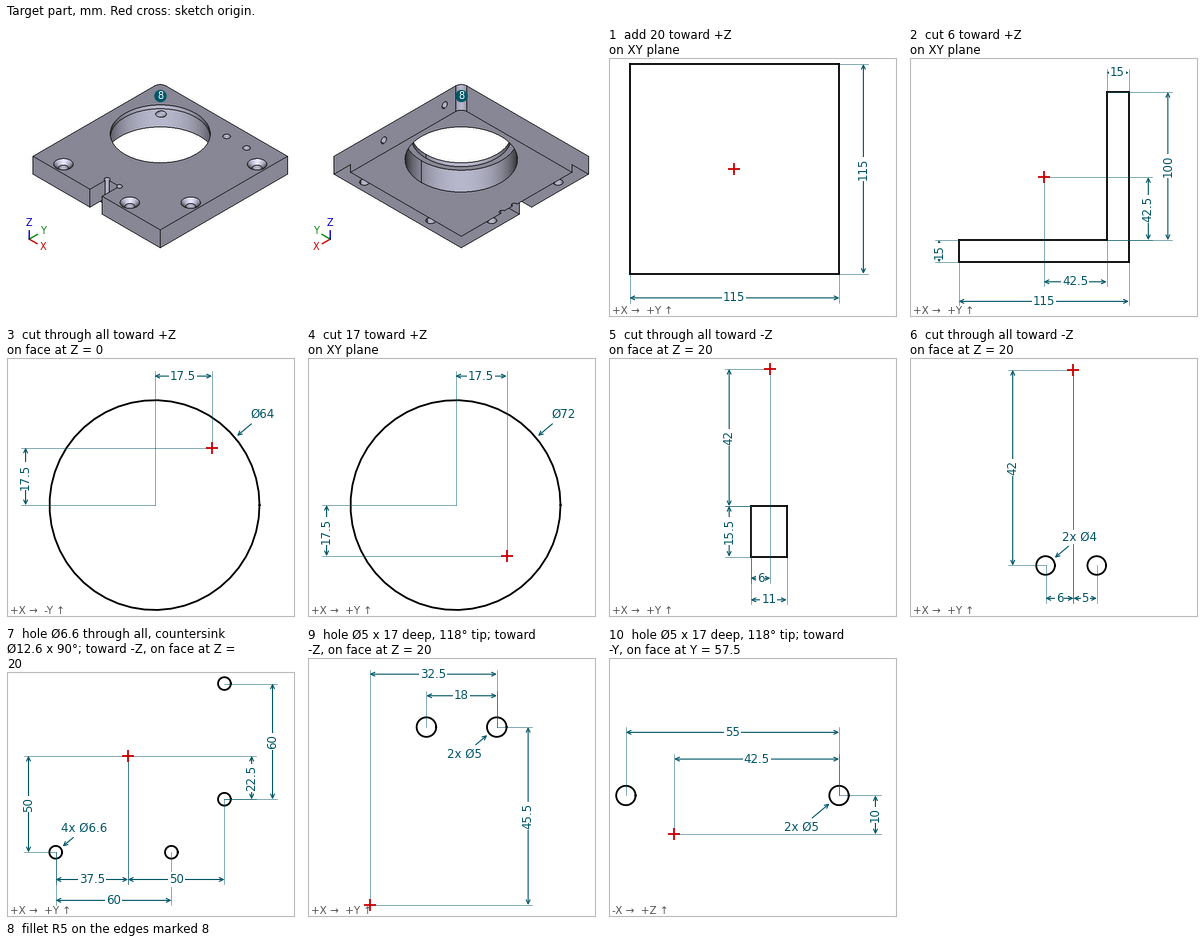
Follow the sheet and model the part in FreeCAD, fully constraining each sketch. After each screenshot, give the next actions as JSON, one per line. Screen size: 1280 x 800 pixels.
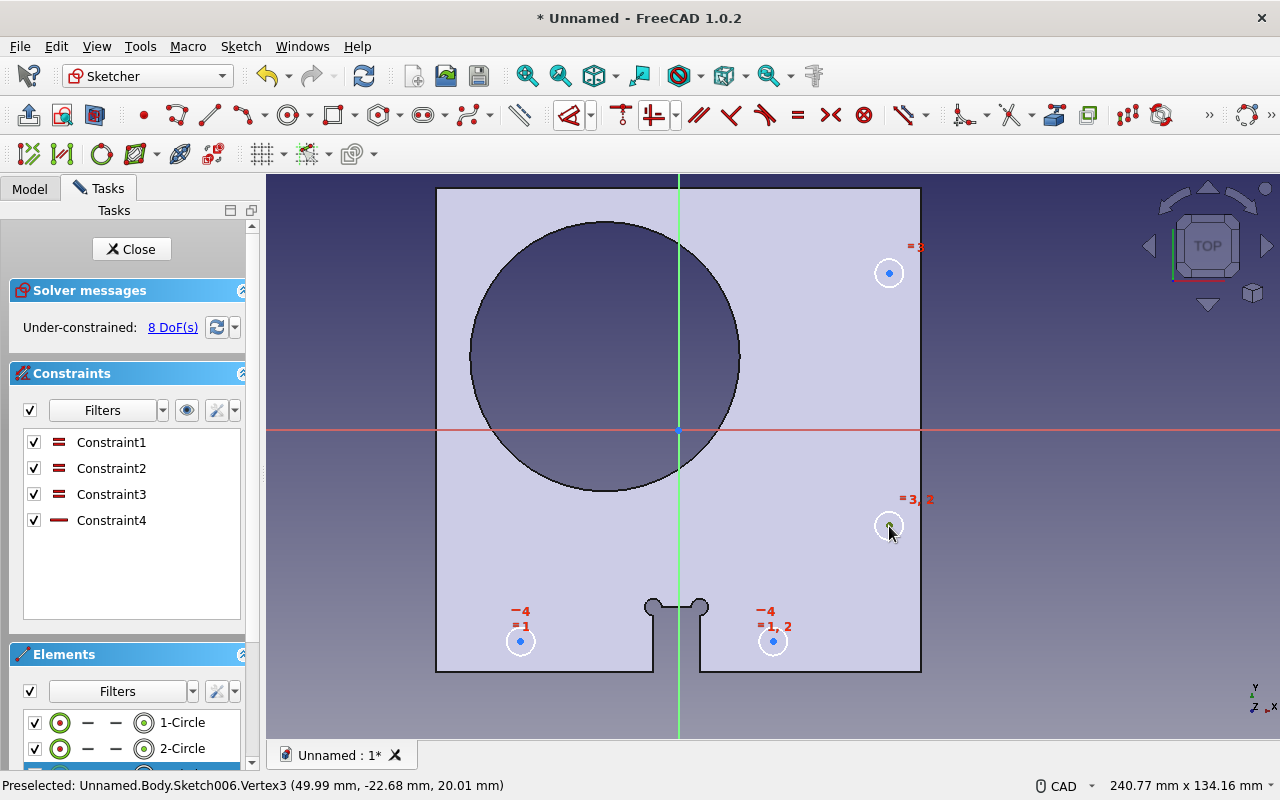
{"action": "left_click", "coordinate": [889, 273]}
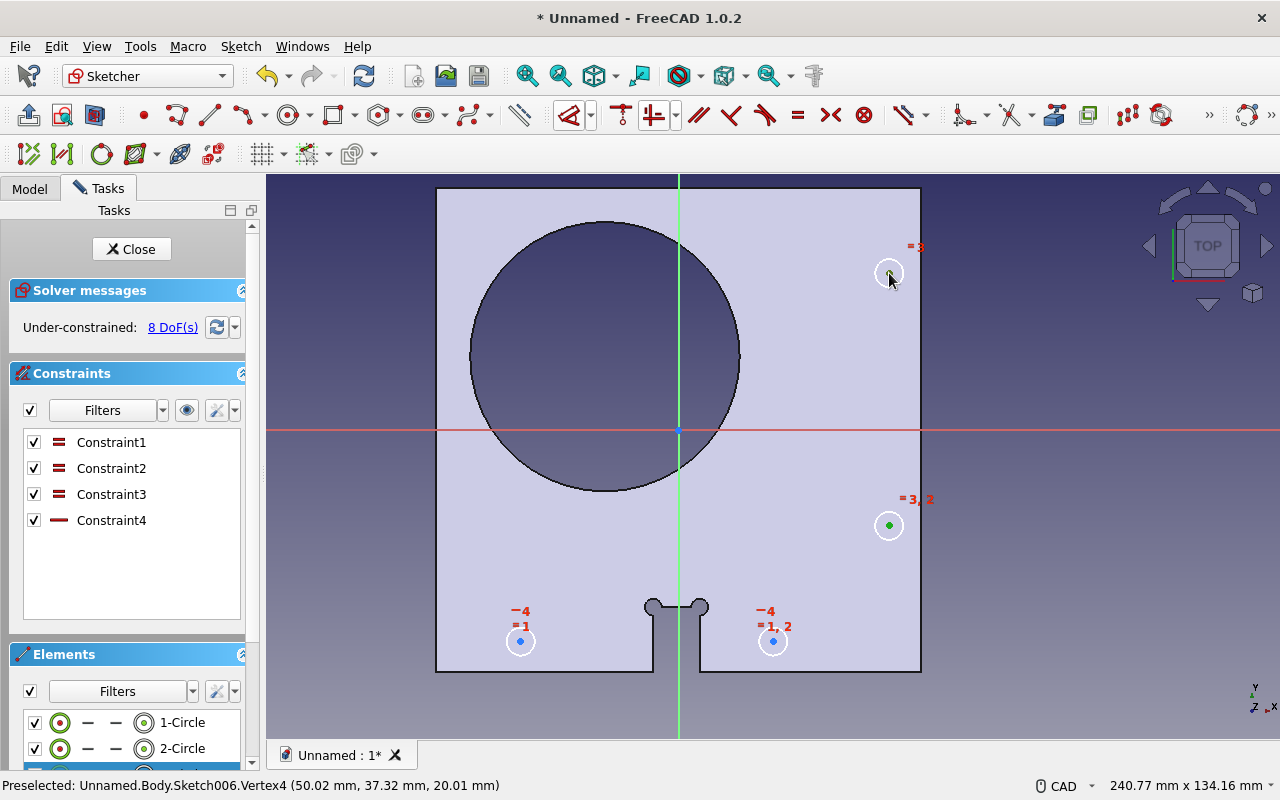
{"action": "key", "text": "v"}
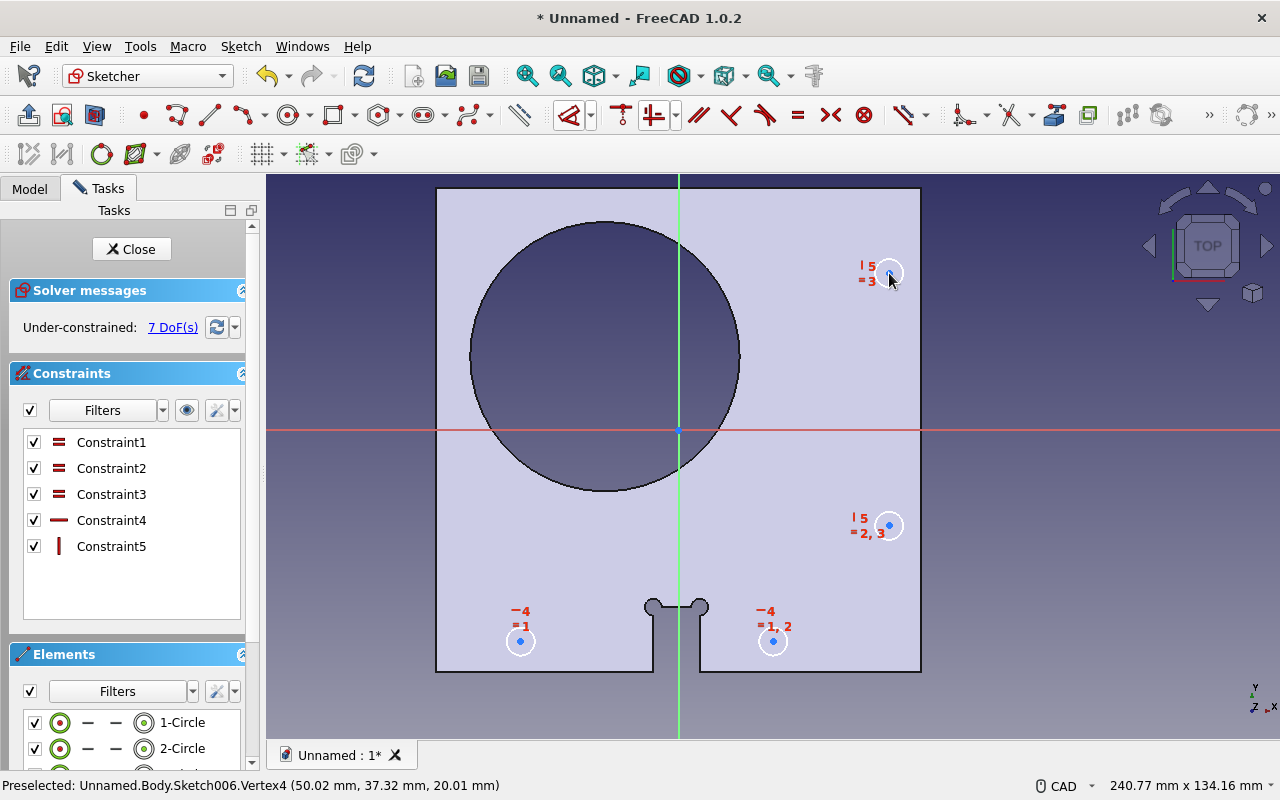
{"action": "scroll", "coordinate": [531, 632], "scroll_direction": "up", "scroll_amount": 2}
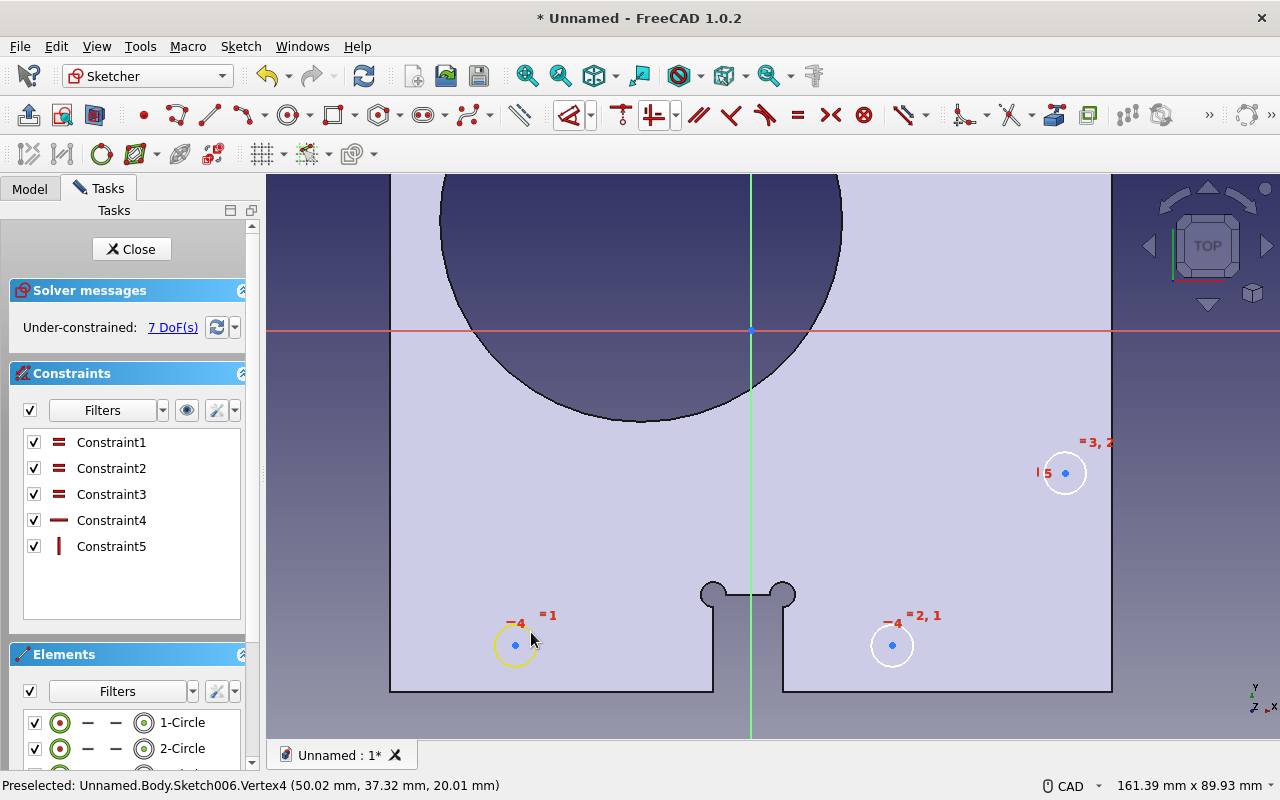
{"action": "left_click", "coordinate": [530, 631]}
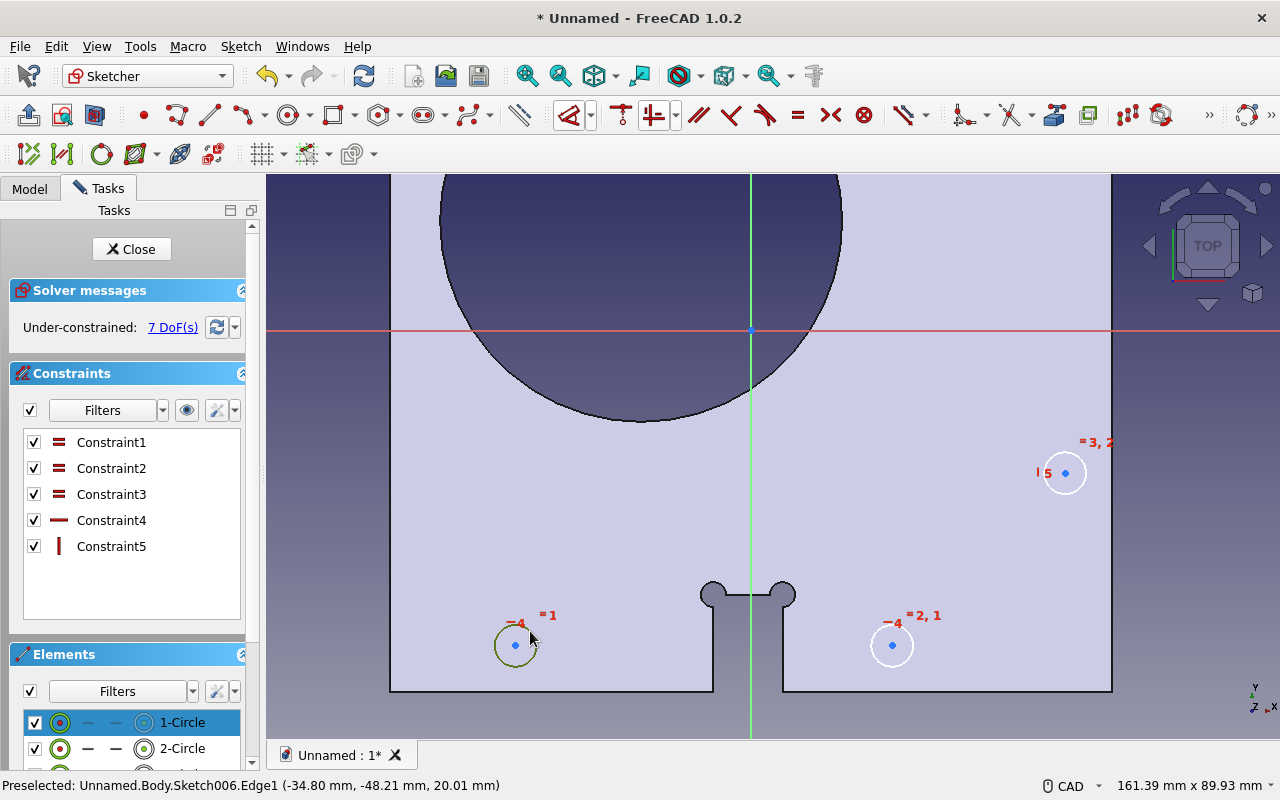
{"action": "key", "text": "k o"}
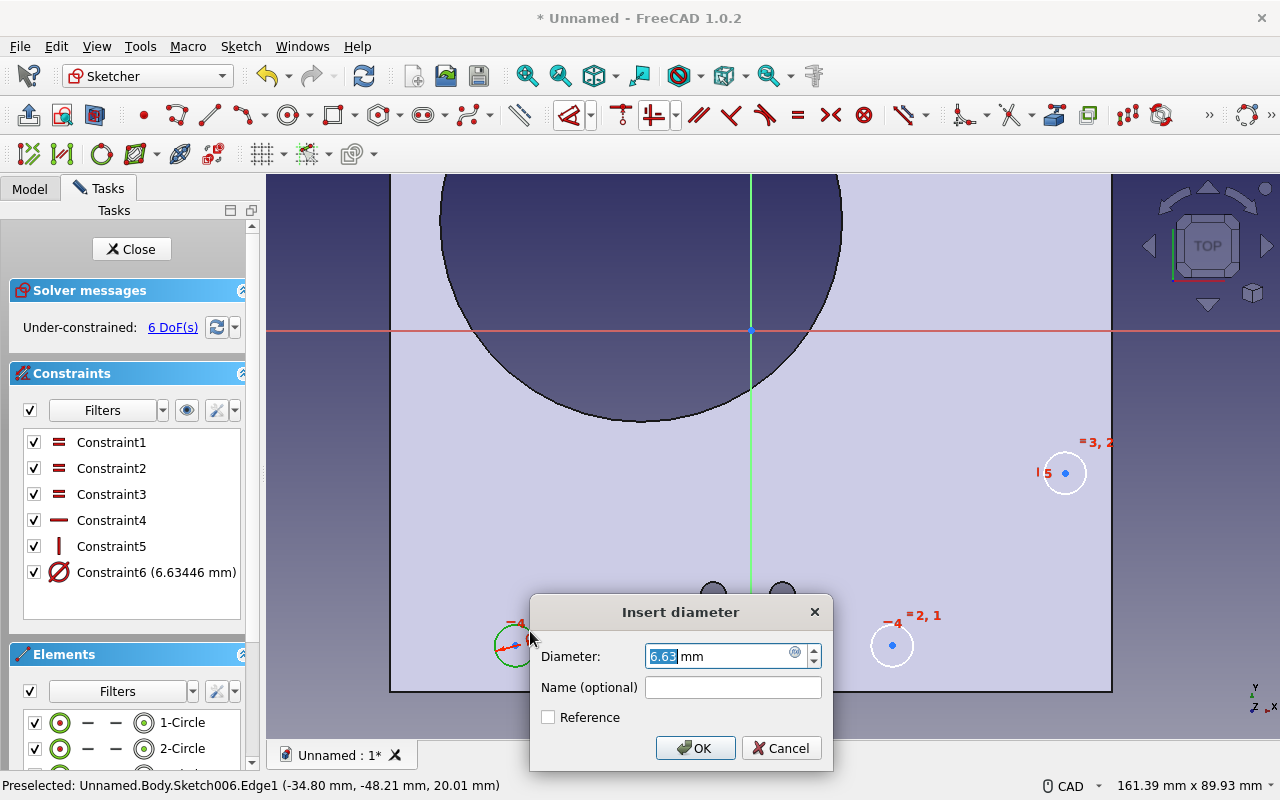
{"action": "type", "text": "6.6"}
{"action": "key", "text": "Return"}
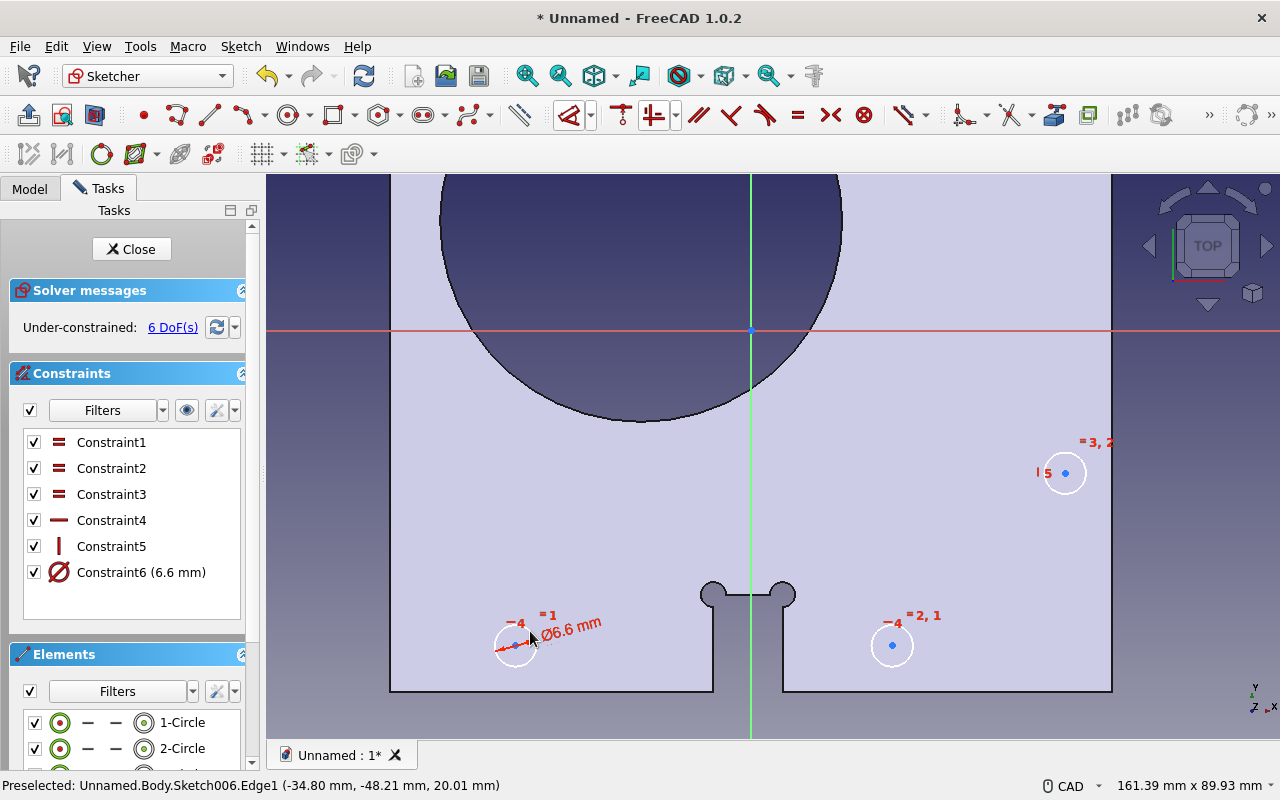
{"action": "left_click", "coordinate": [516, 646]}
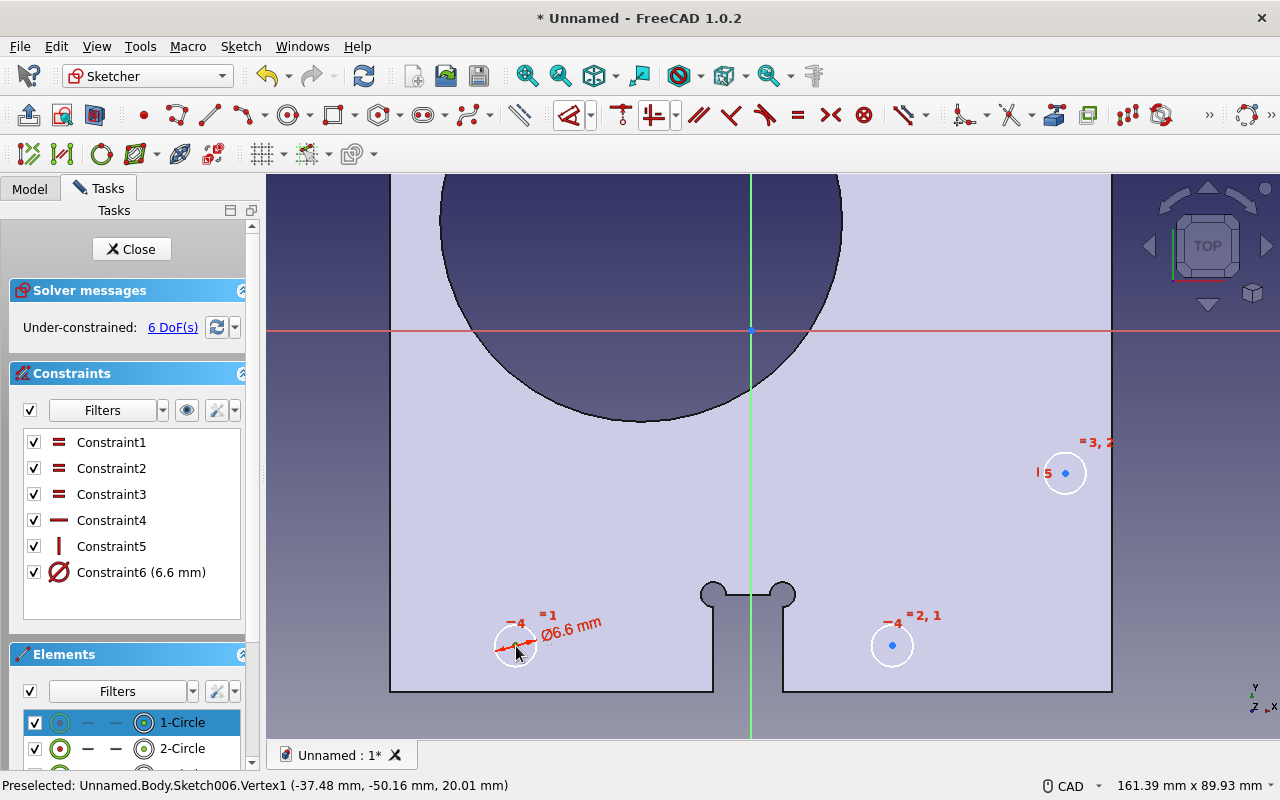
{"action": "key", "text": "i"}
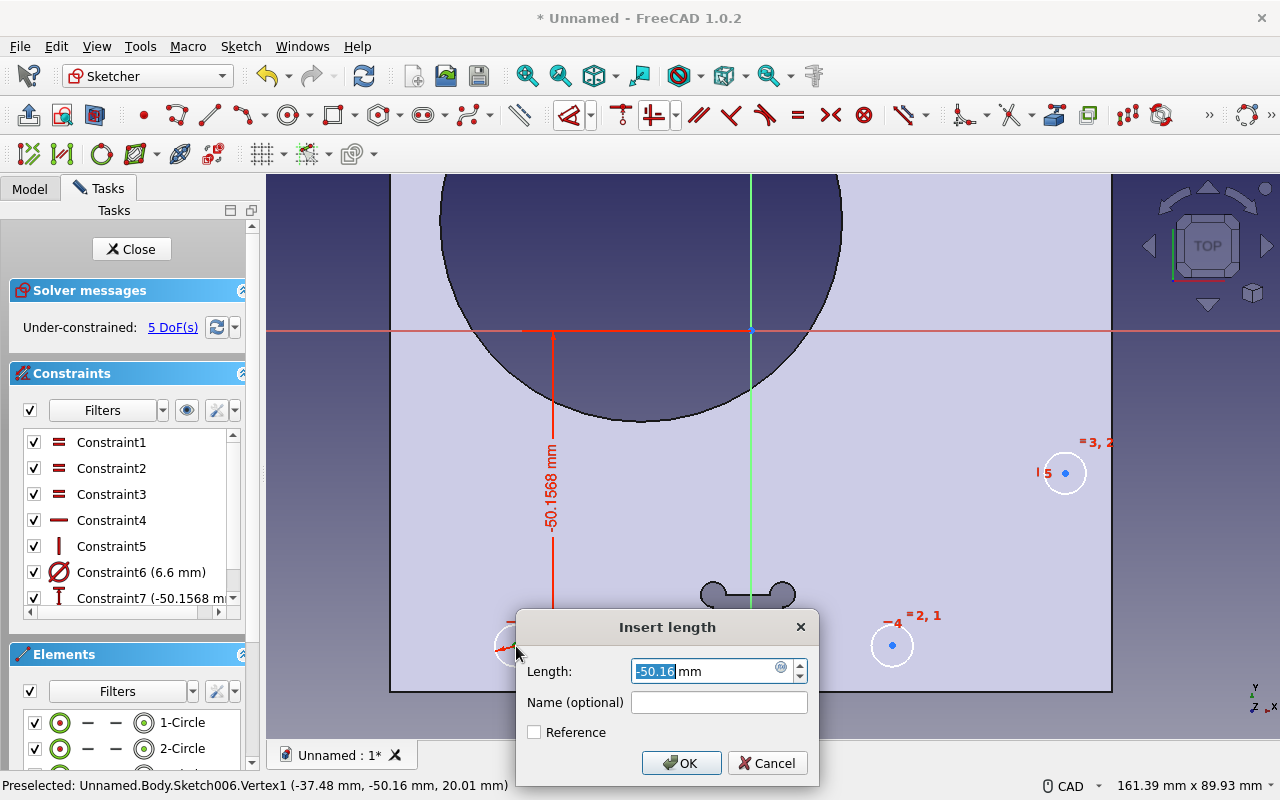
{"action": "type", "text": "-50"}
{"action": "key", "text": "Return"}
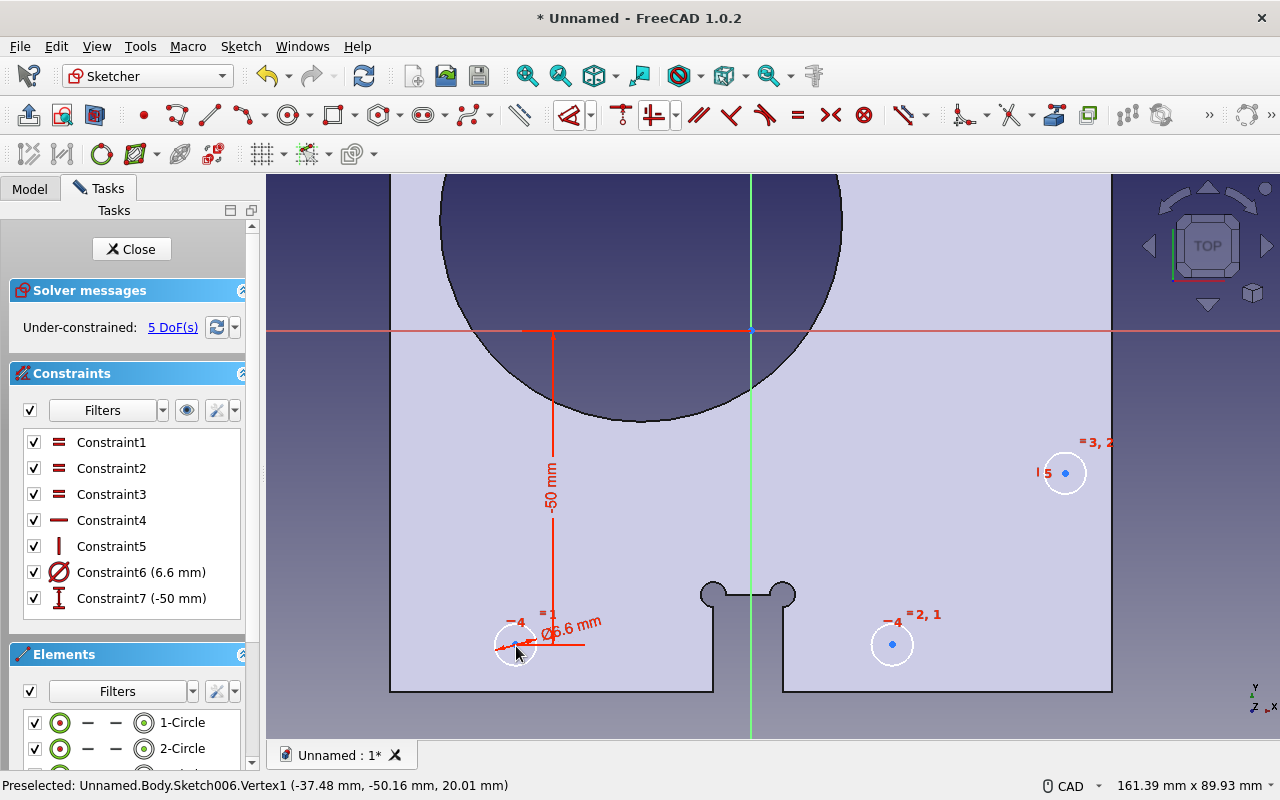
{"action": "left_click", "coordinate": [1065, 473]}